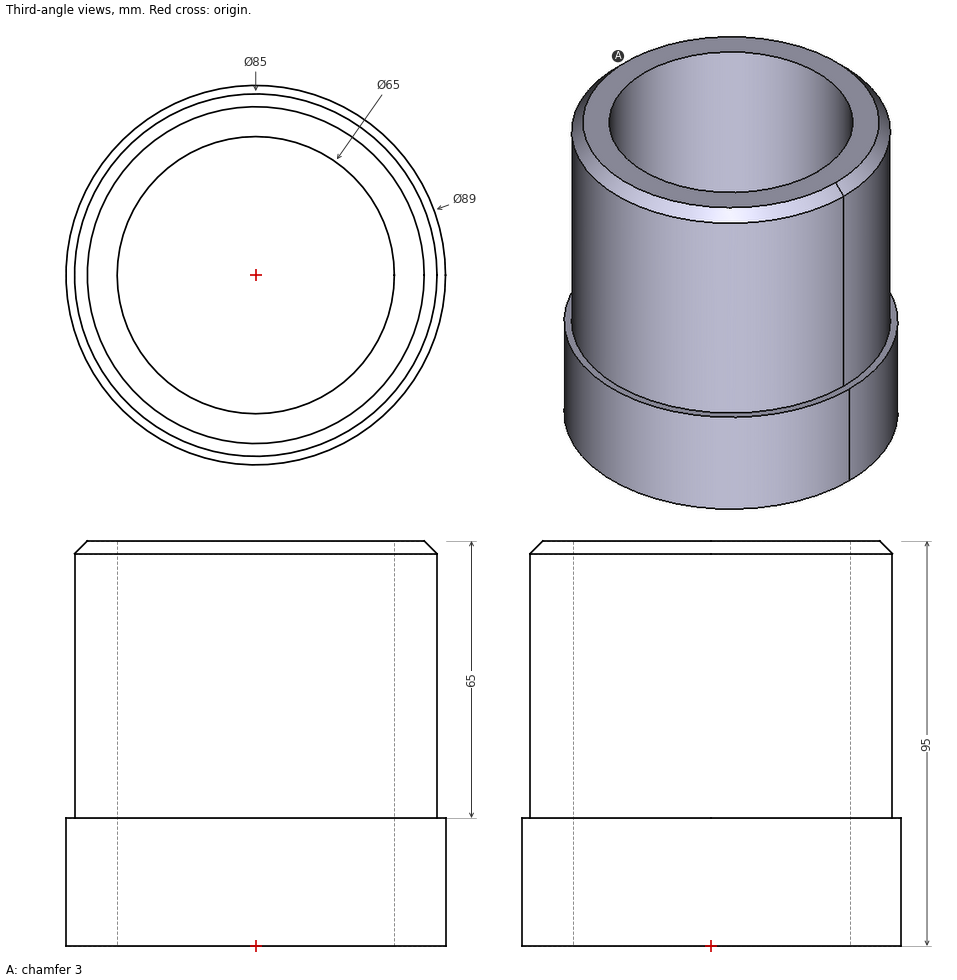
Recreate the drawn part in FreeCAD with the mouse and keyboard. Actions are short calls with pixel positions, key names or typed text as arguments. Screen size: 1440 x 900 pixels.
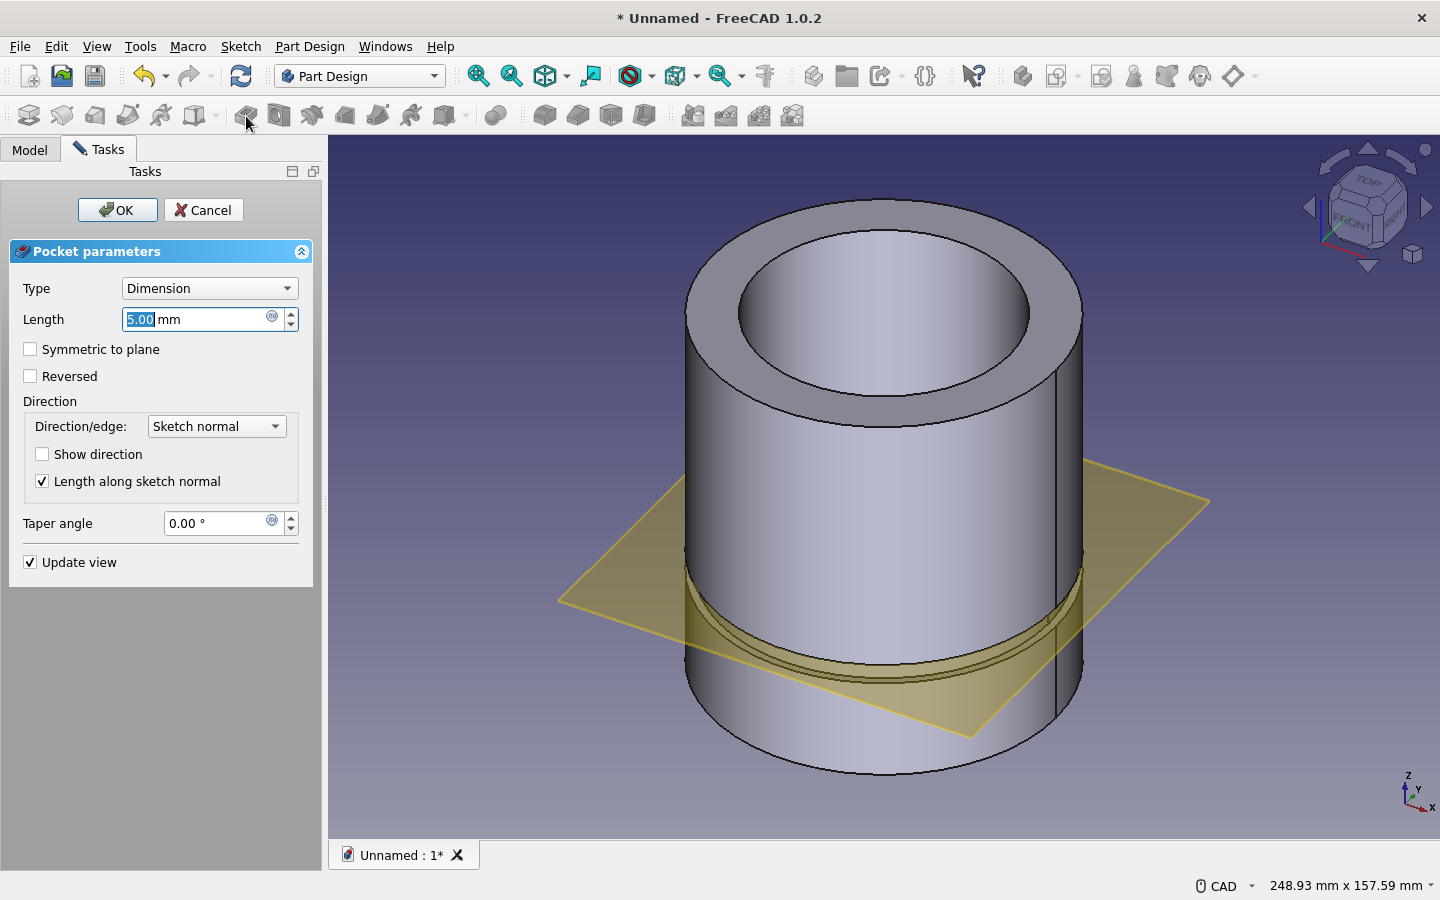
text(65)
key(Tab)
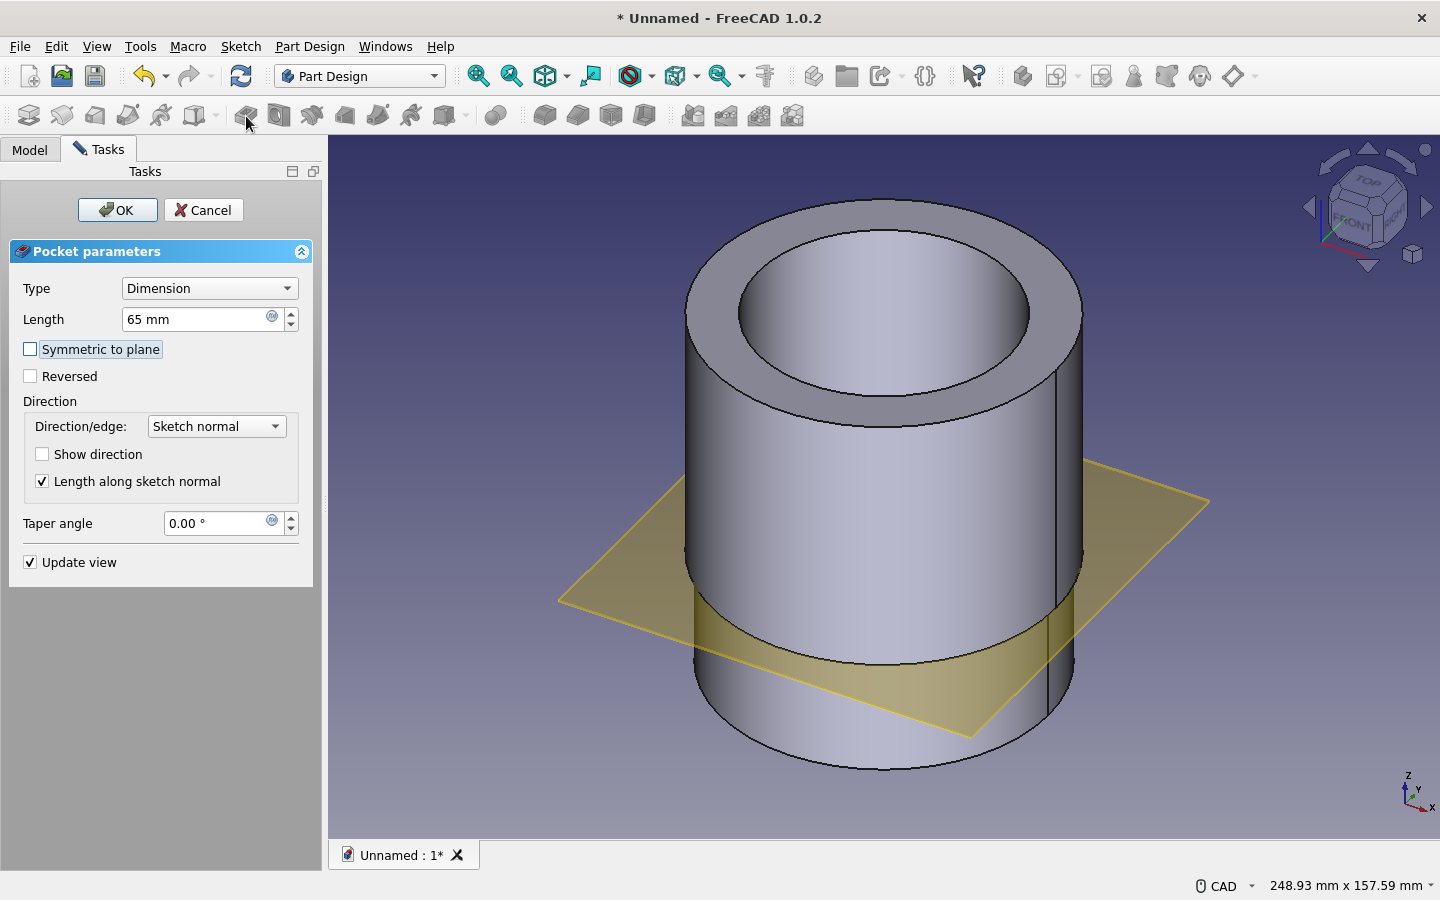
click(31, 376)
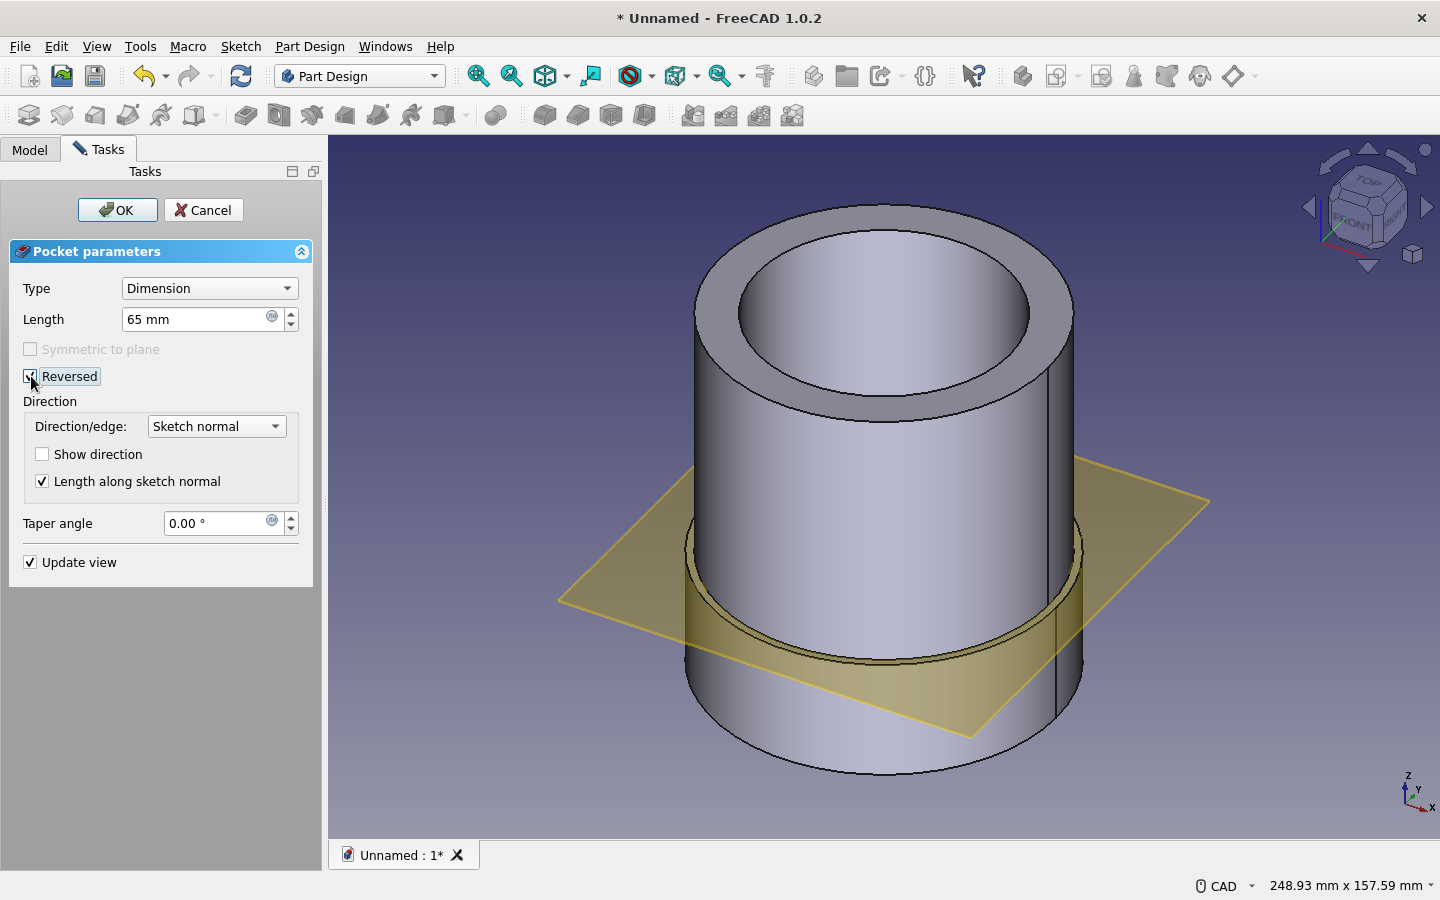
click(118, 210)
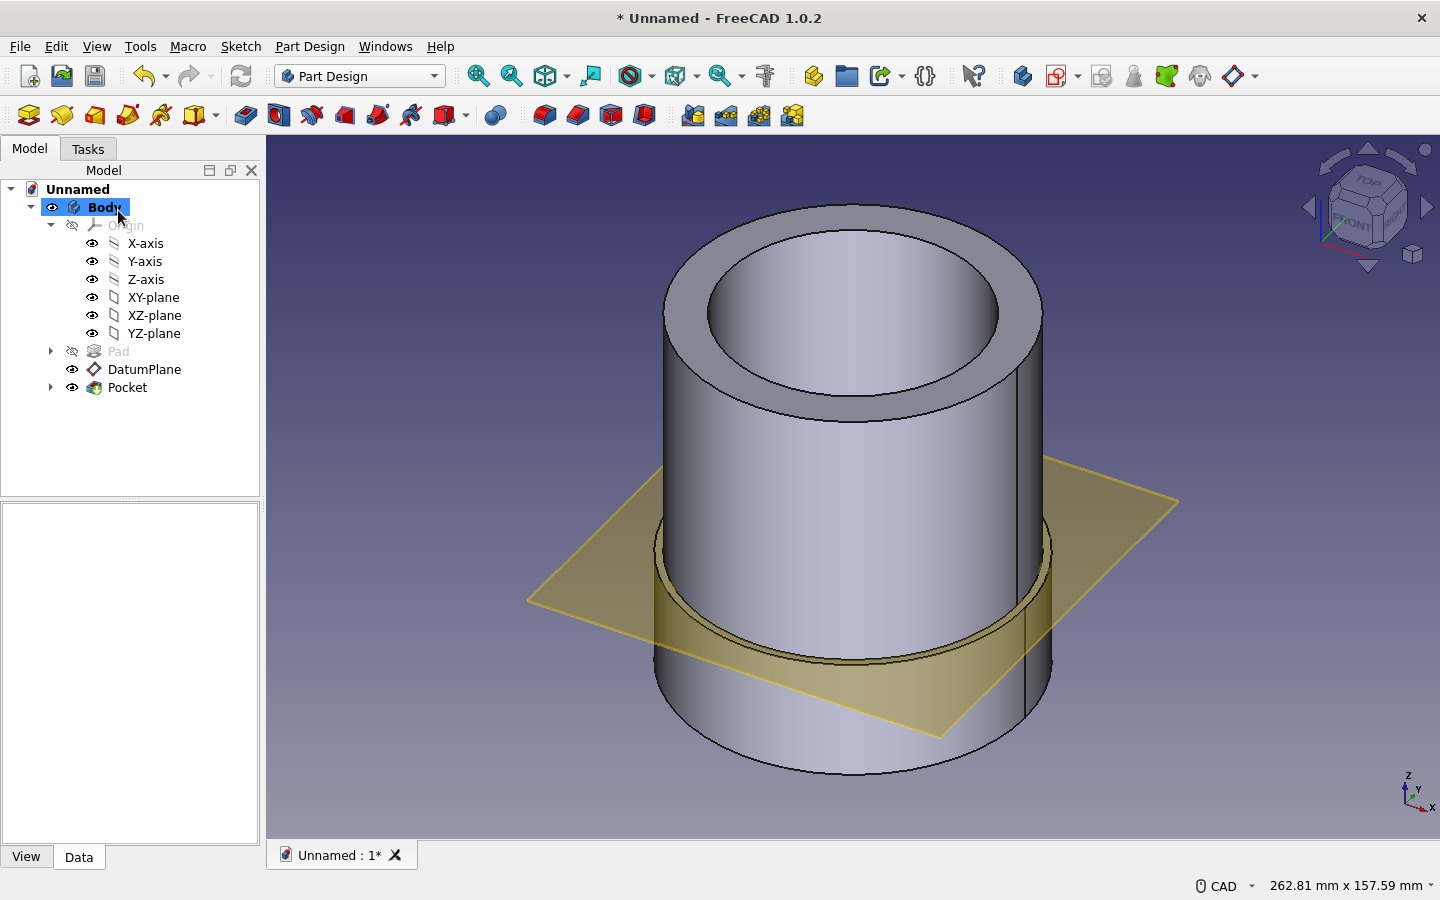
click(117, 369)
key(space)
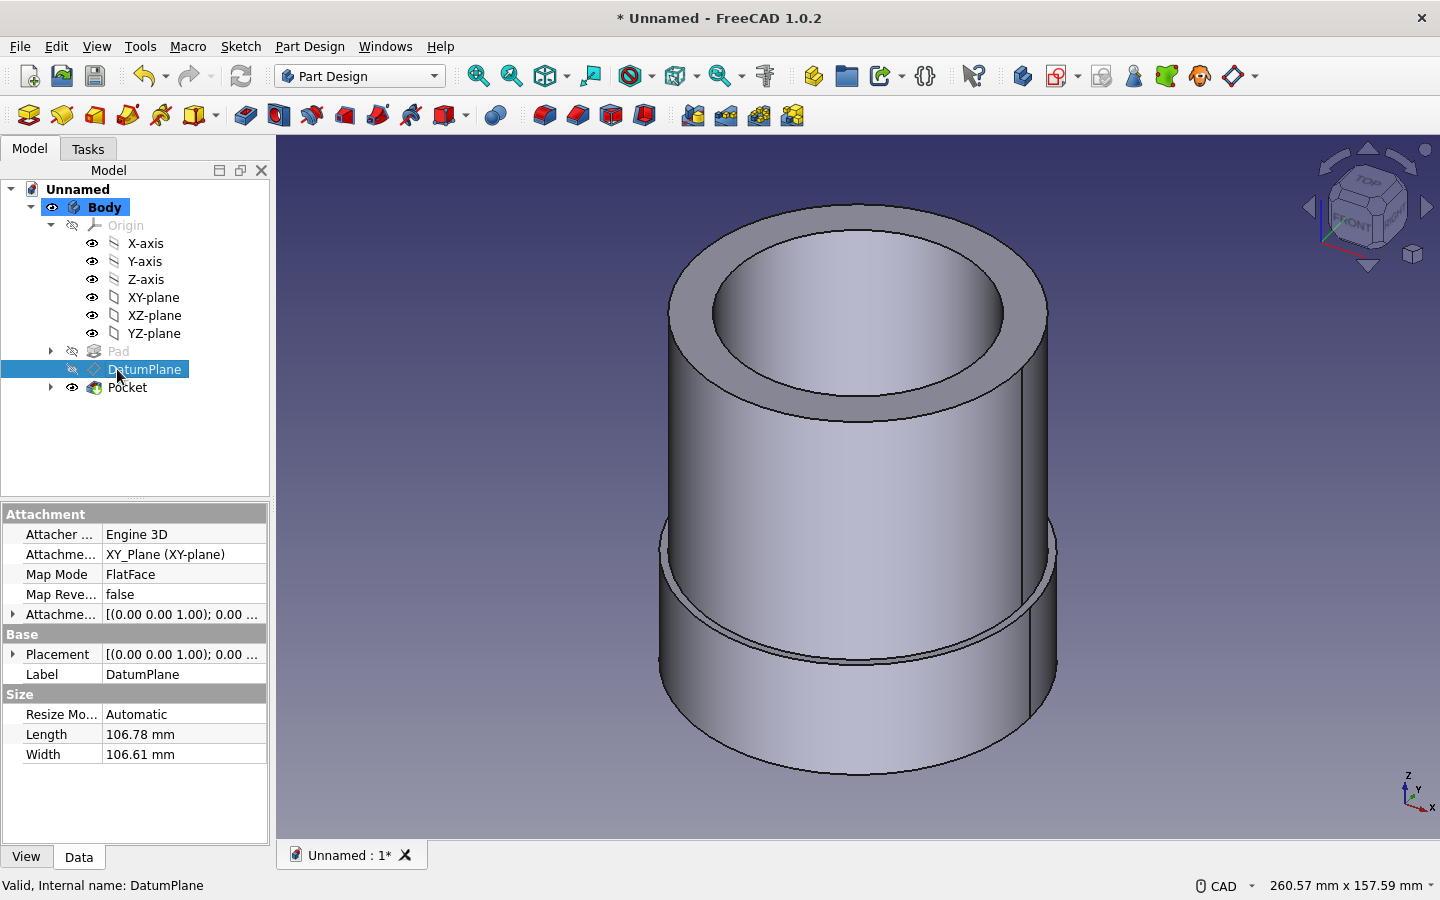
click(669, 324)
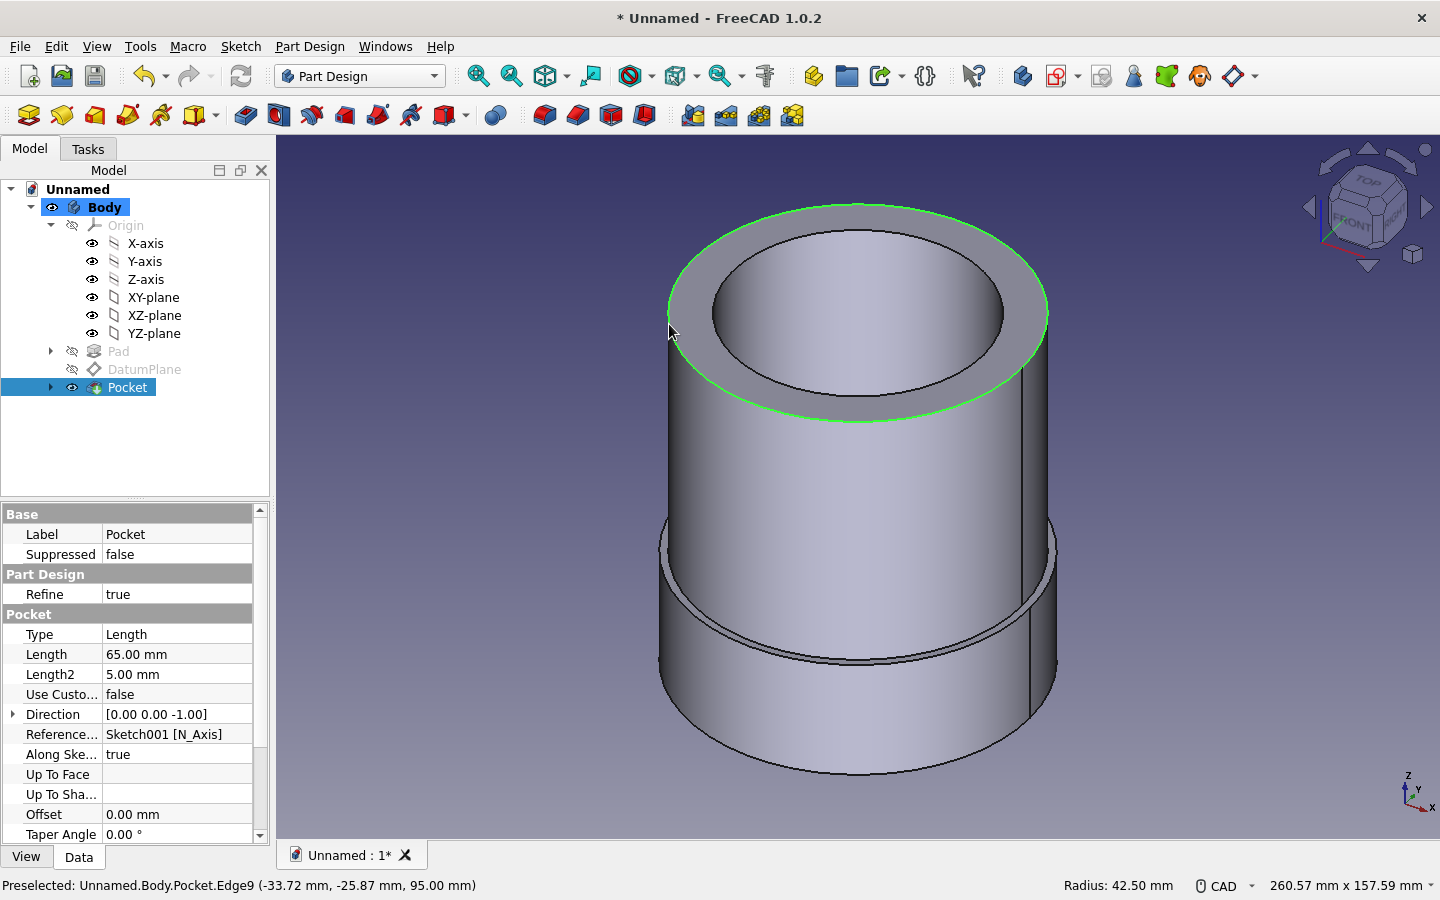
click(578, 116)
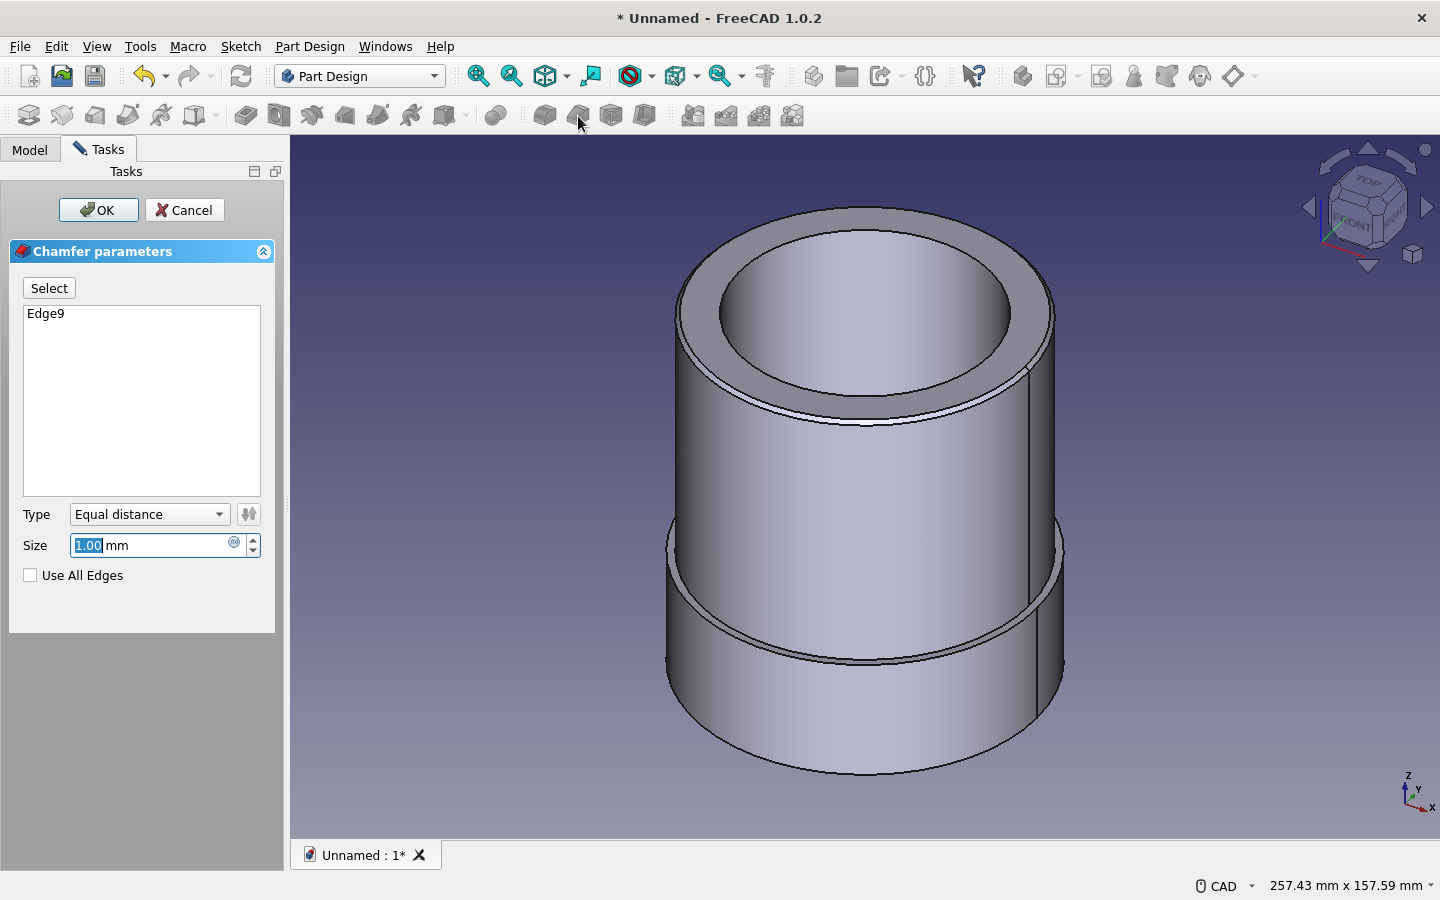
text(3)
key(Tab)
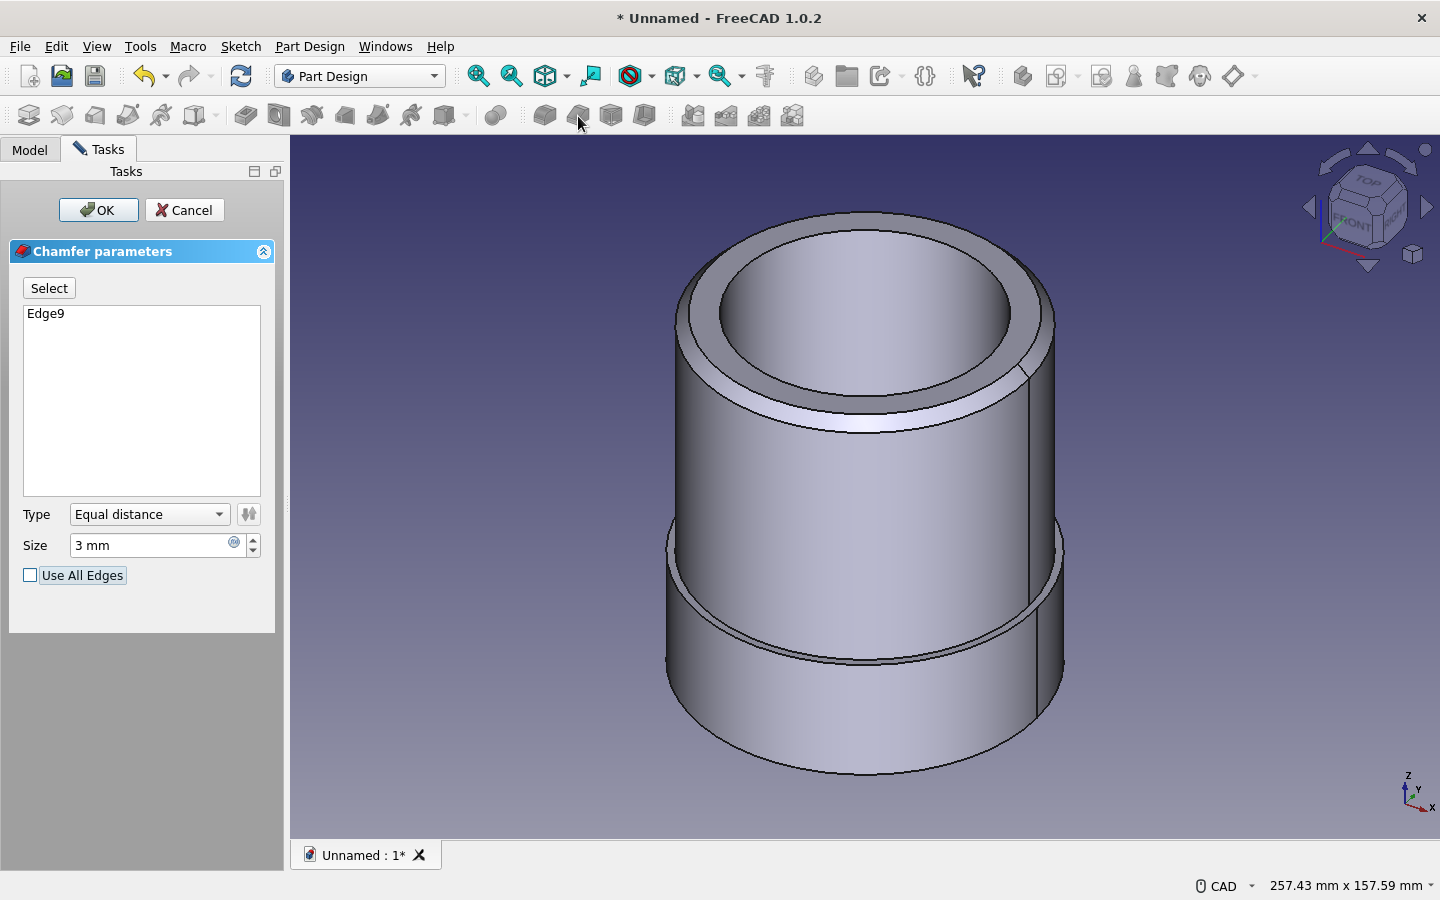
click(99, 210)